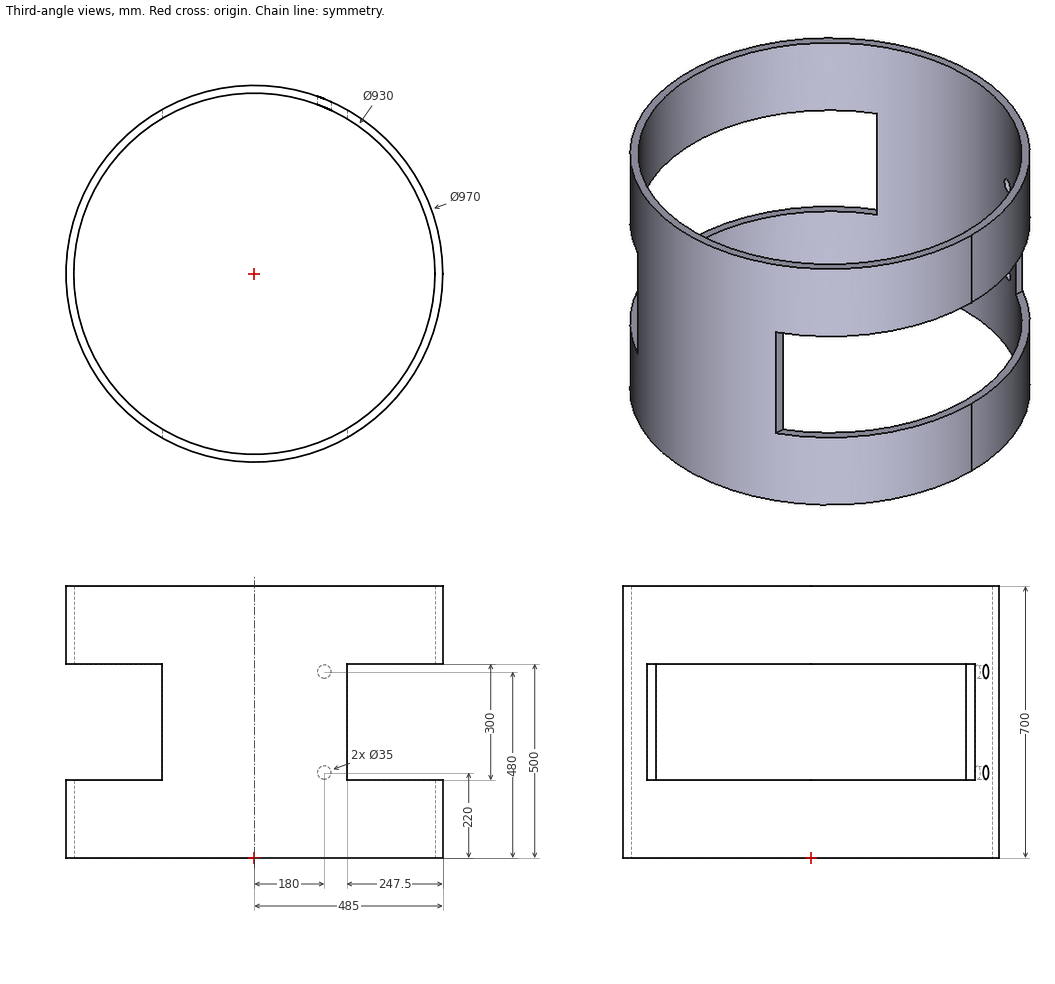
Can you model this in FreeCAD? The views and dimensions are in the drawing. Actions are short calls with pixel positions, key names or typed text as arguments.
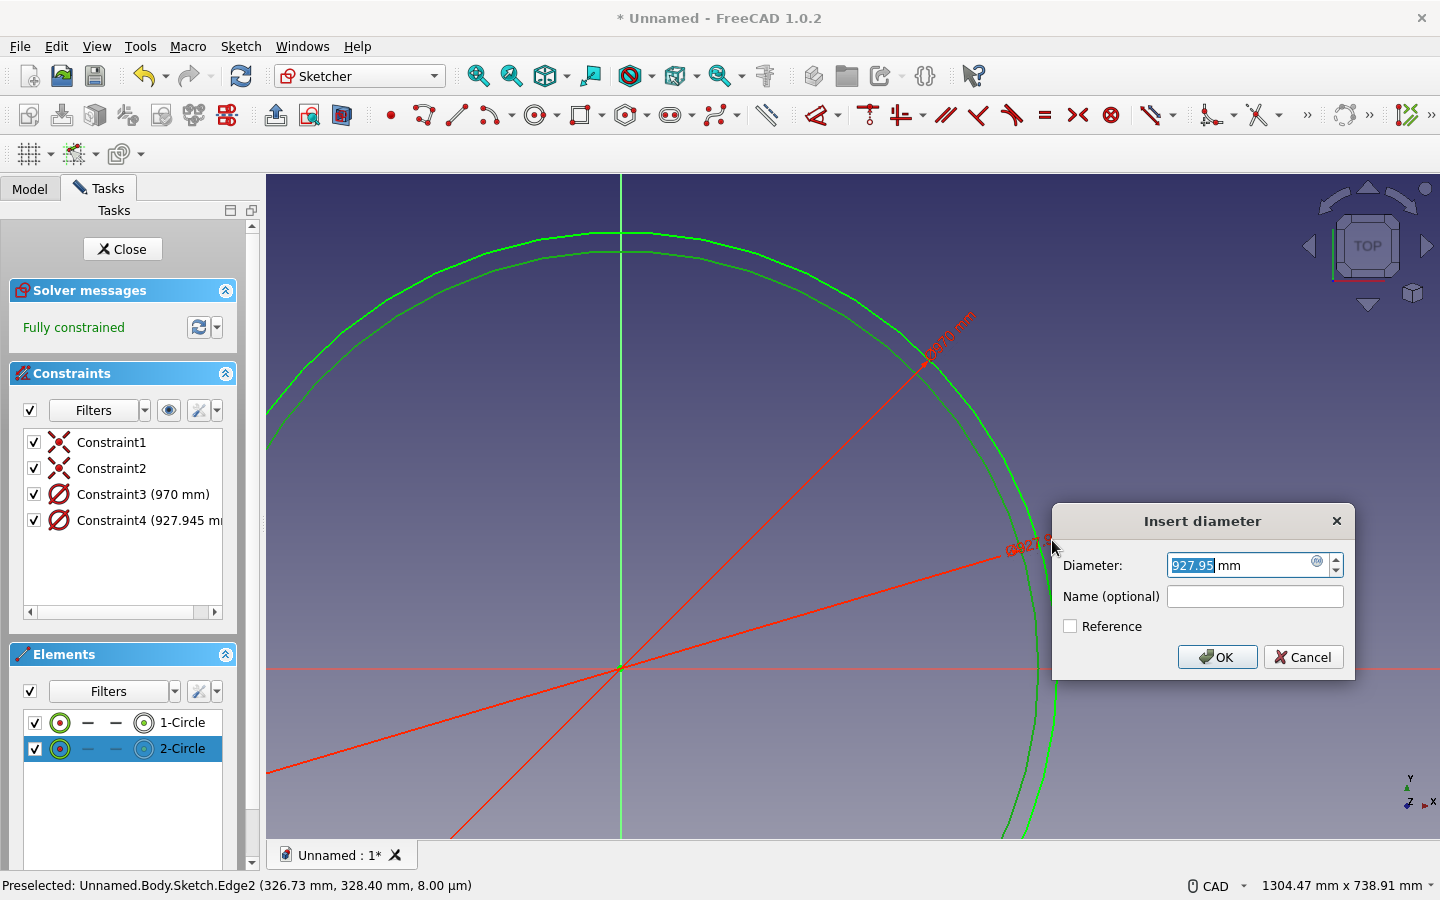
text(930)
key(Return)
key(Escape)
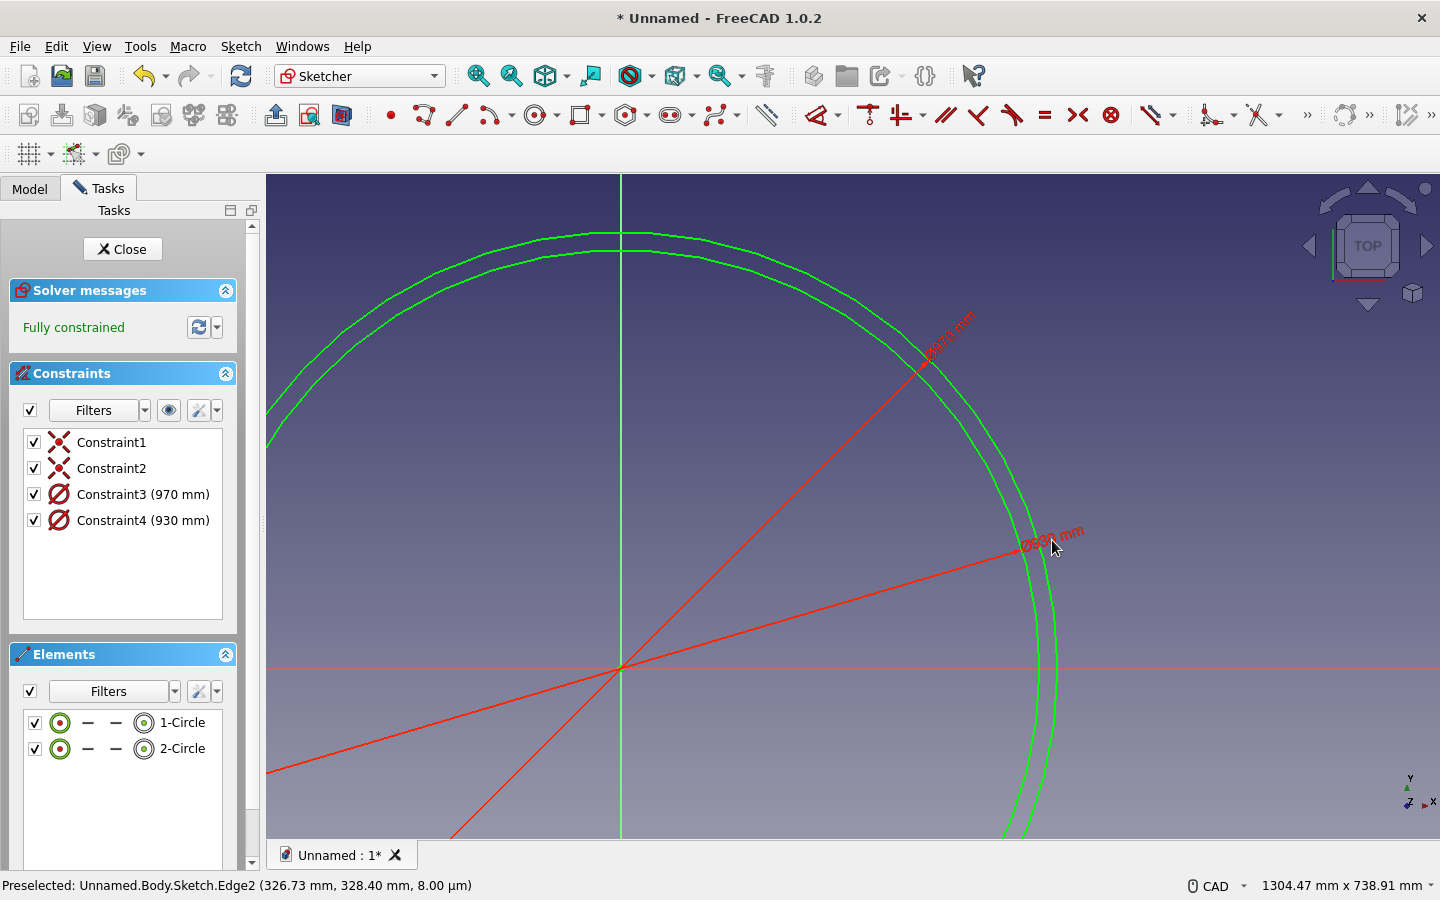
click(123, 249)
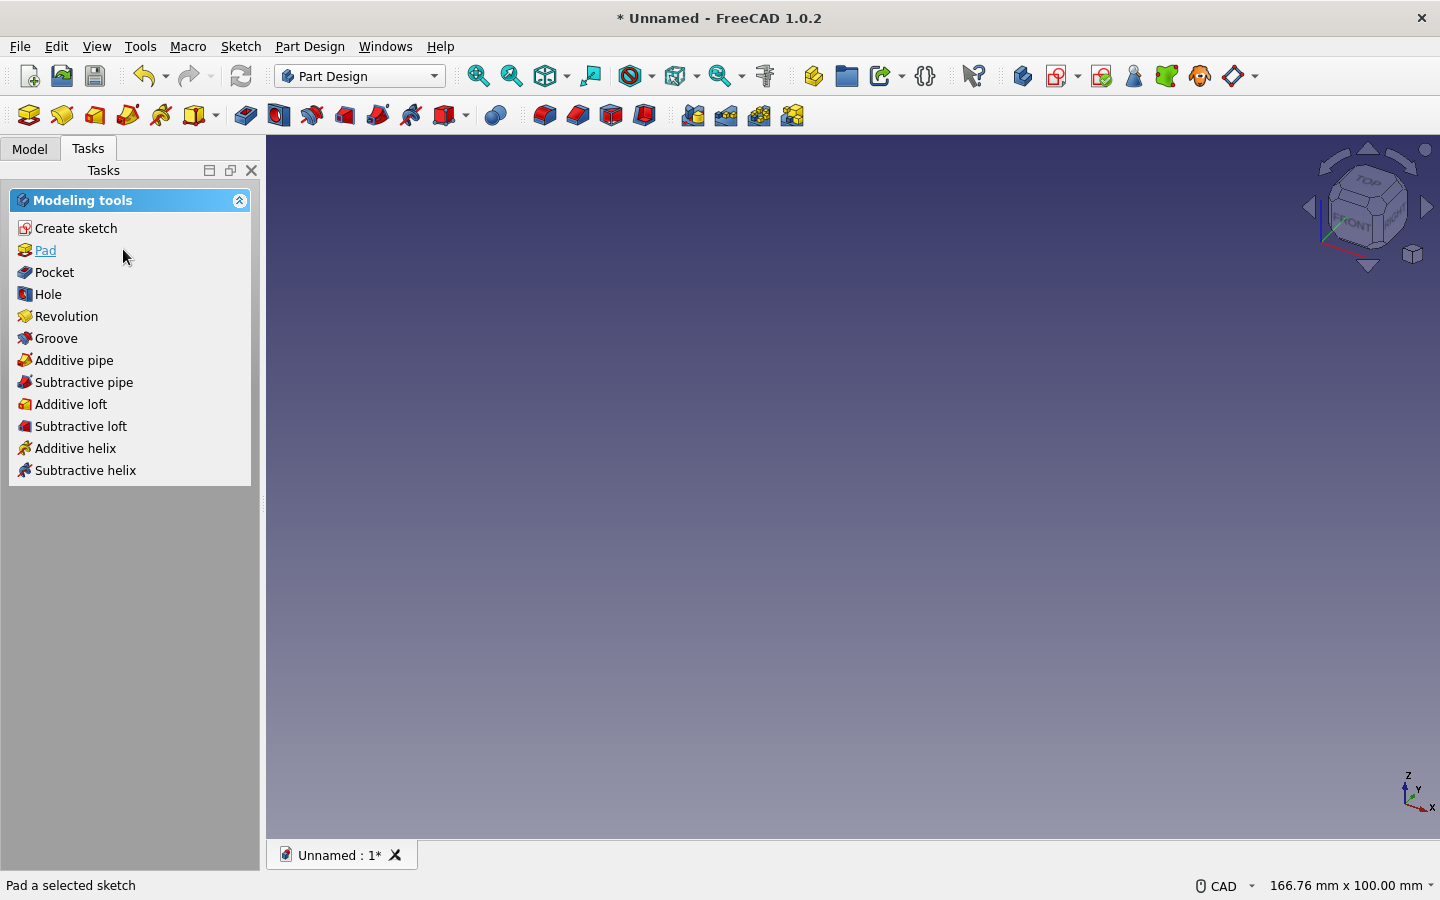
click(29, 116)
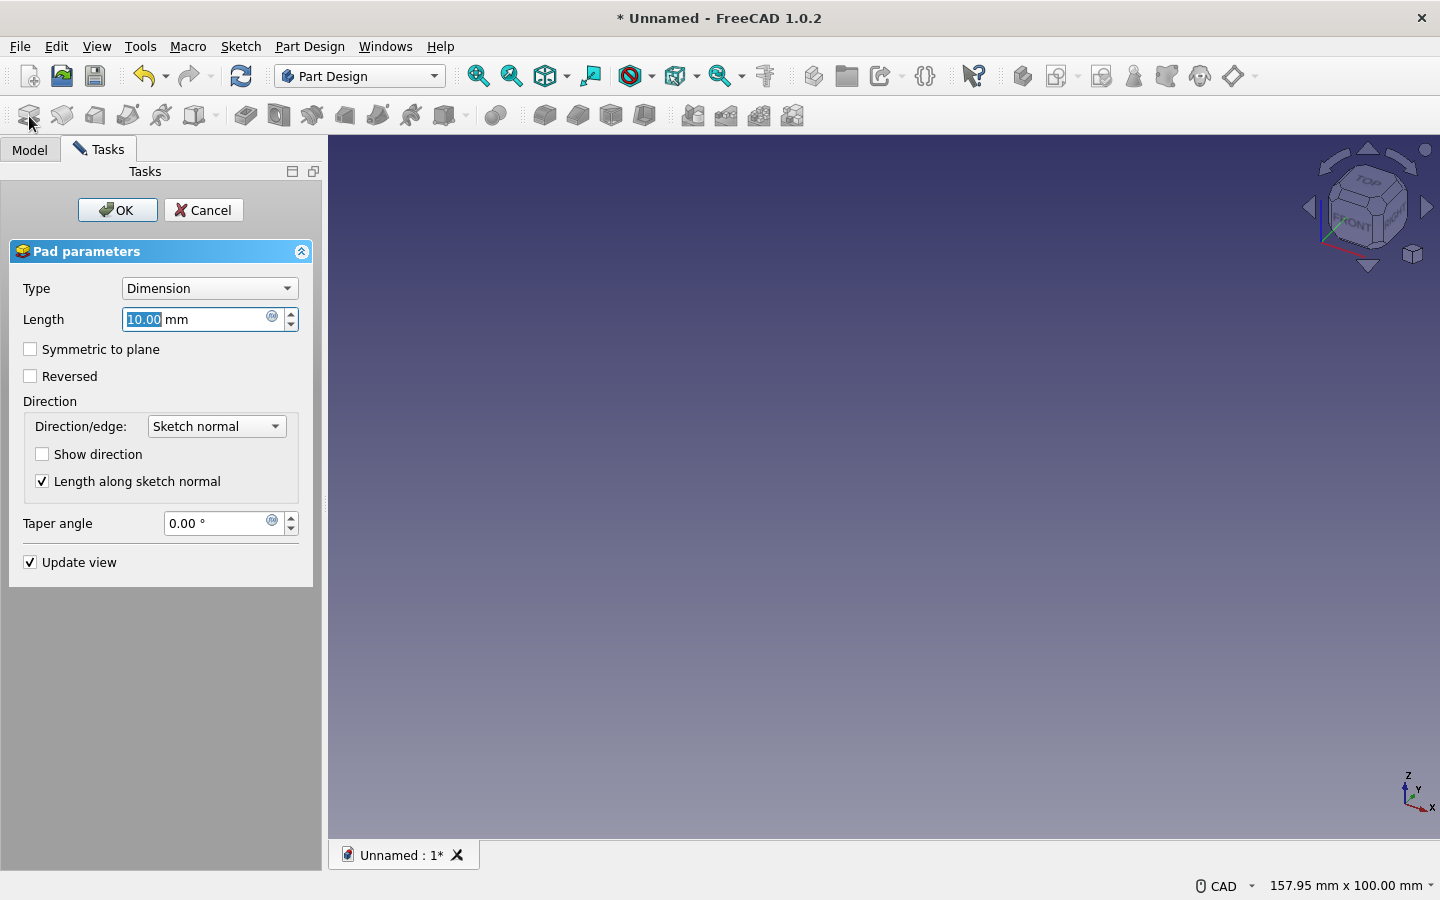
text(700)
key(Tab)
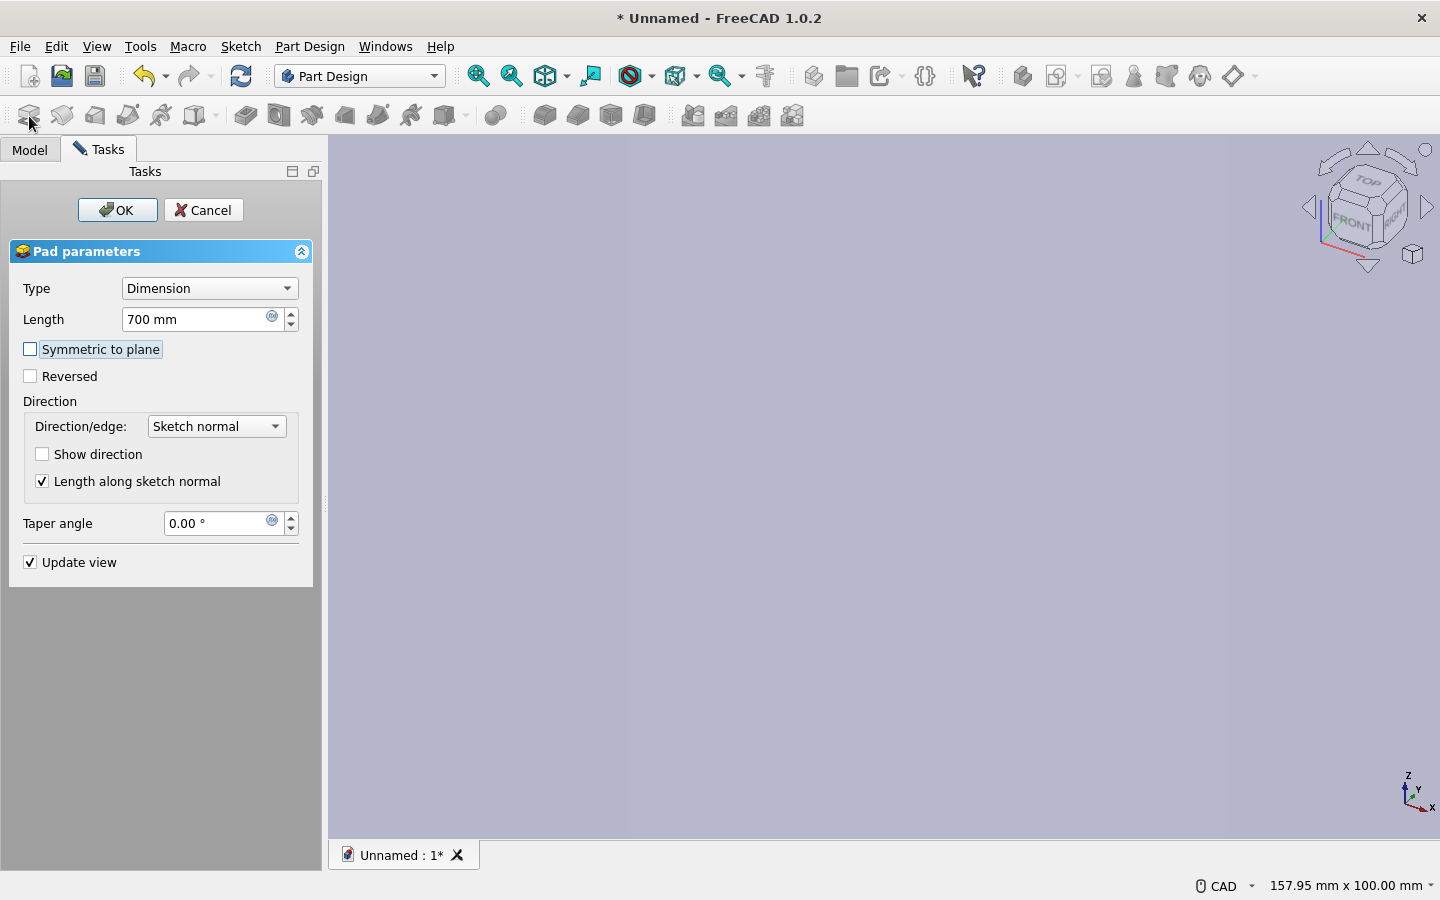
click(118, 210)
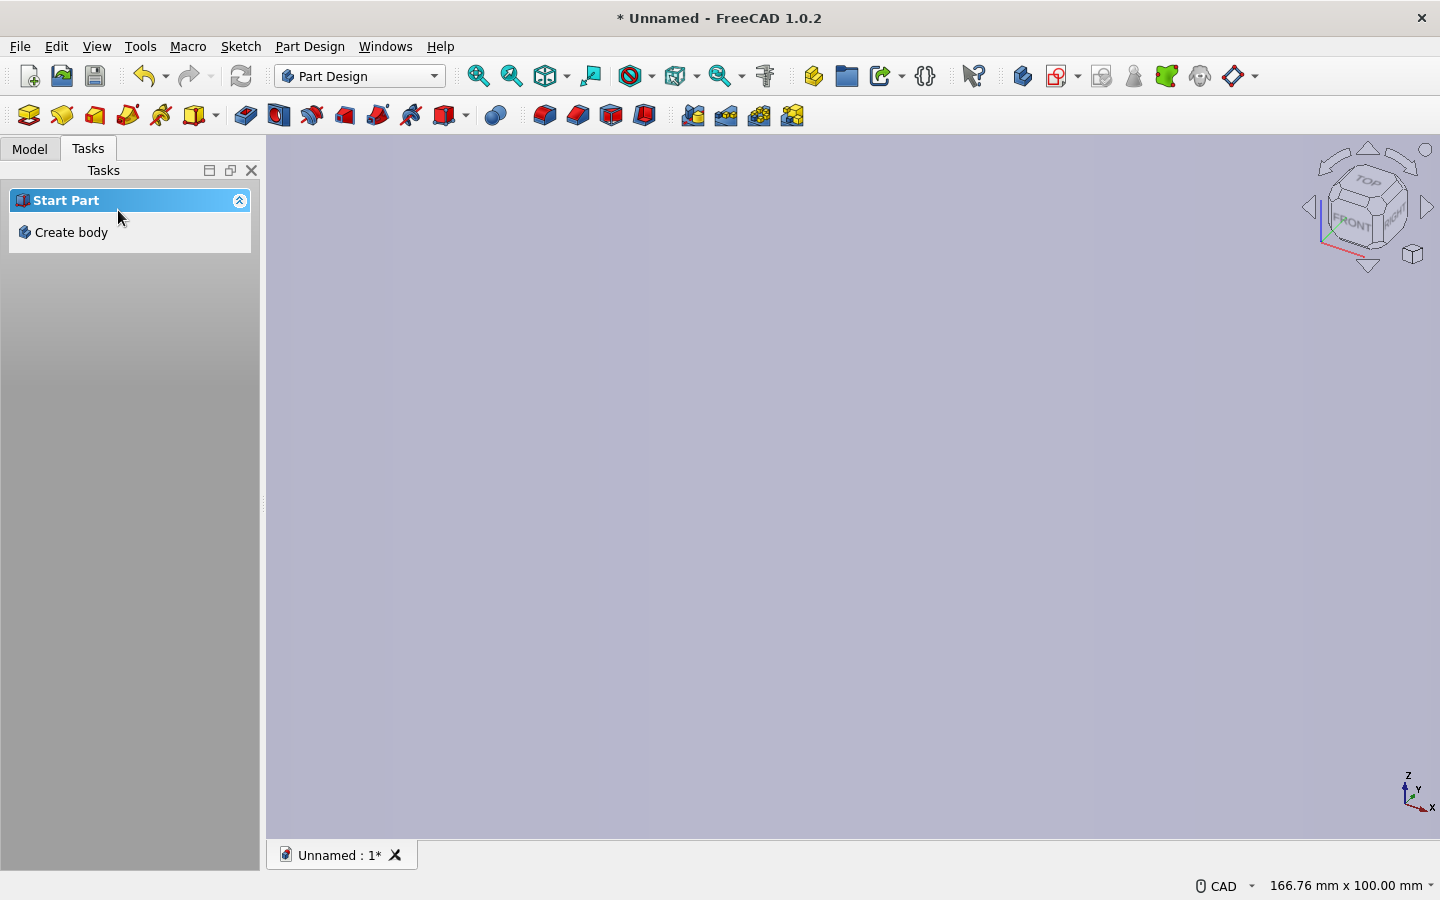
key(v)
key(f)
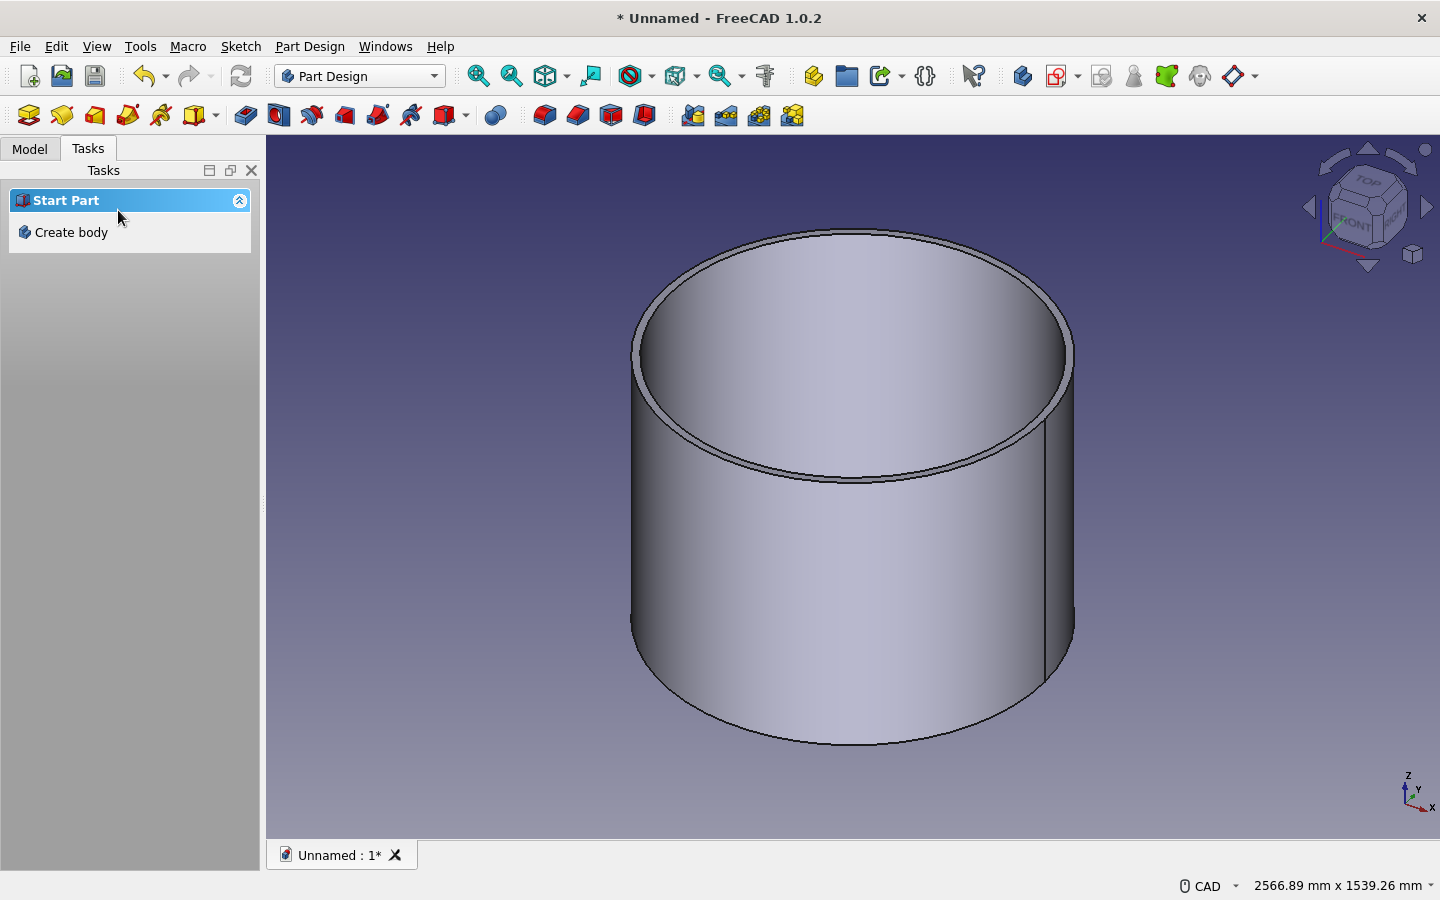
click(1056, 76)